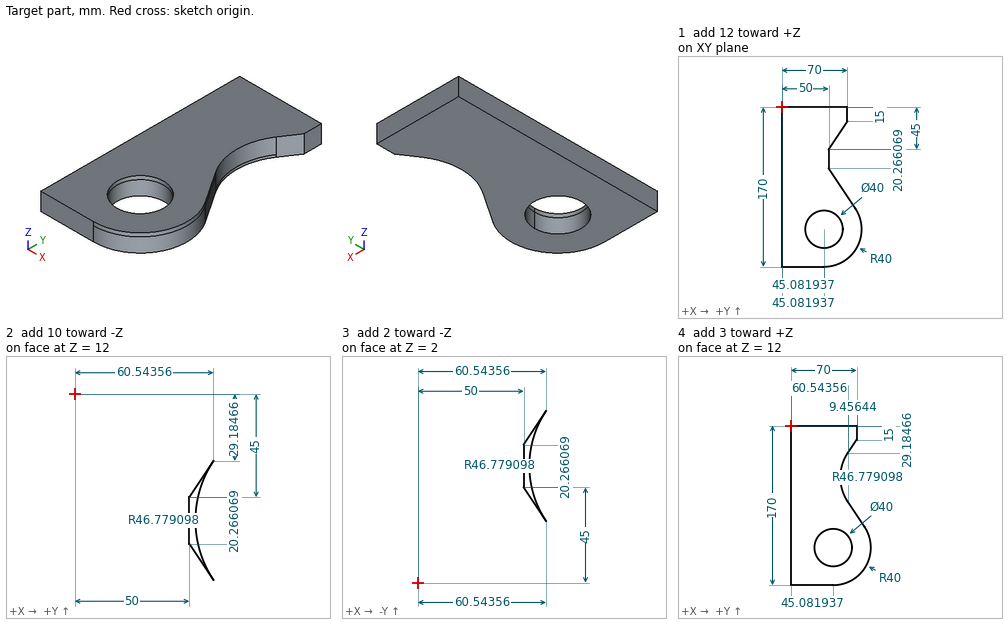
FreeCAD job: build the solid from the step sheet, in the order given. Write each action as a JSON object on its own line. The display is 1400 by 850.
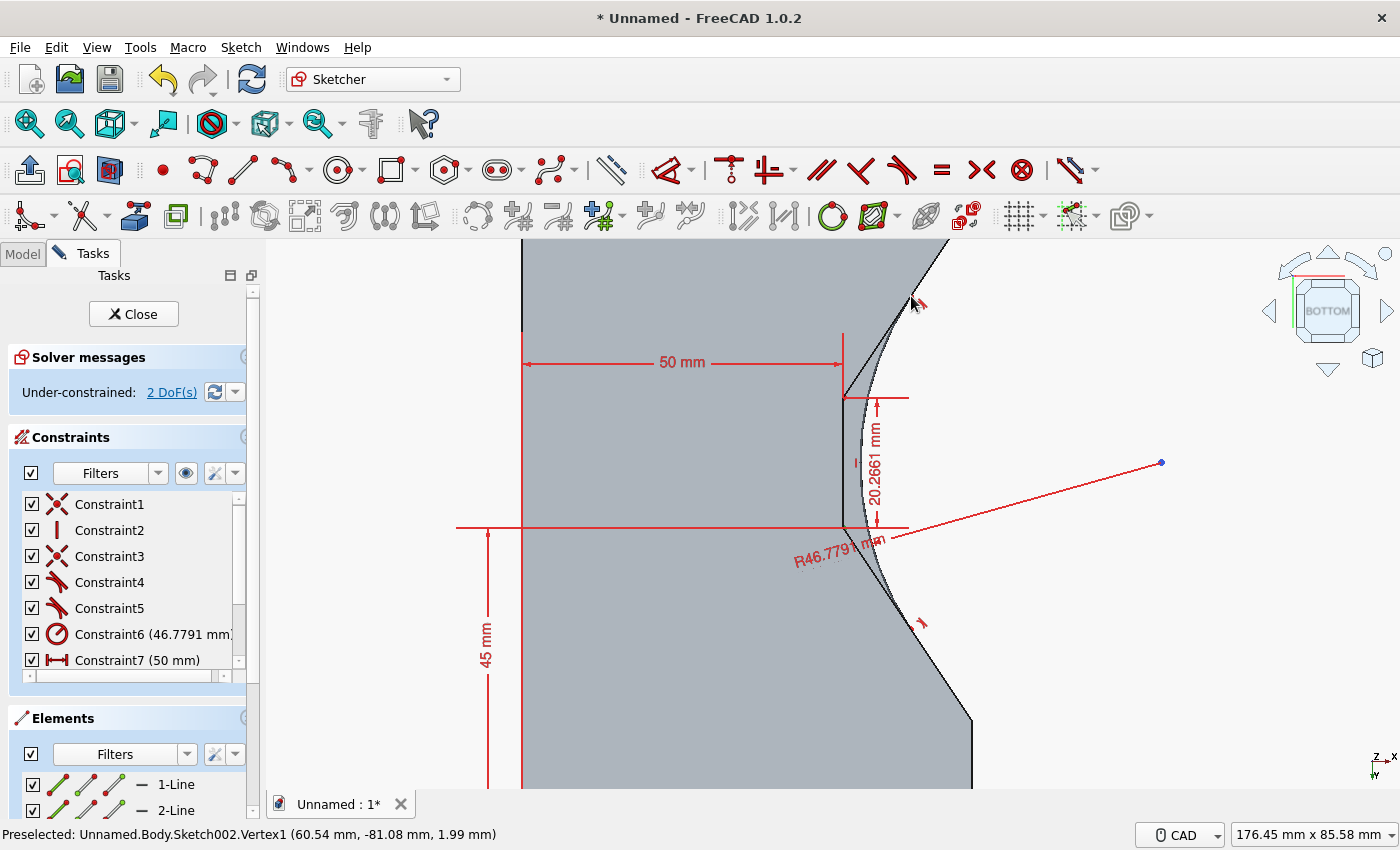
{"action": "left_click", "coordinate": [911, 296]}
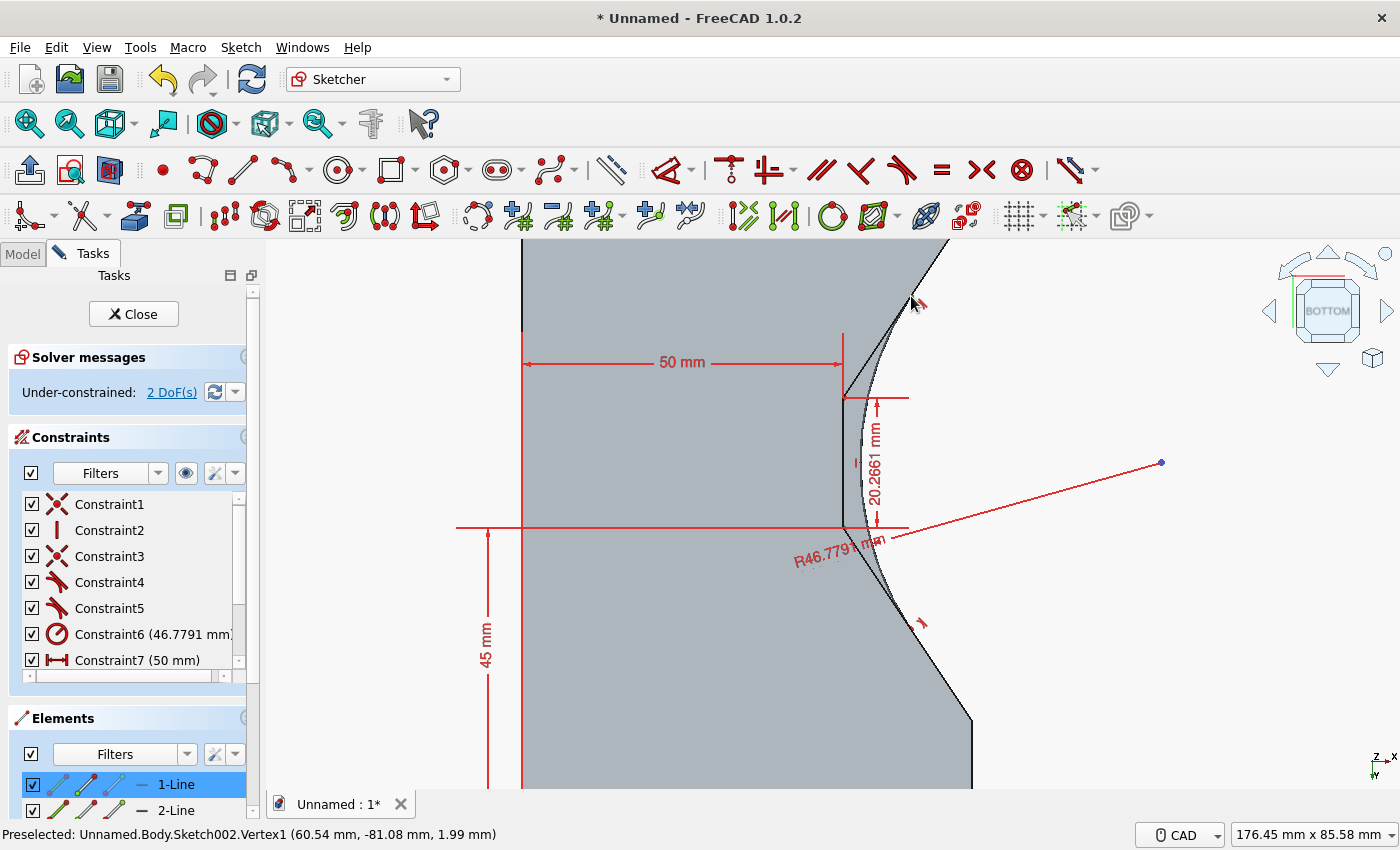
{"action": "key", "text": "l"}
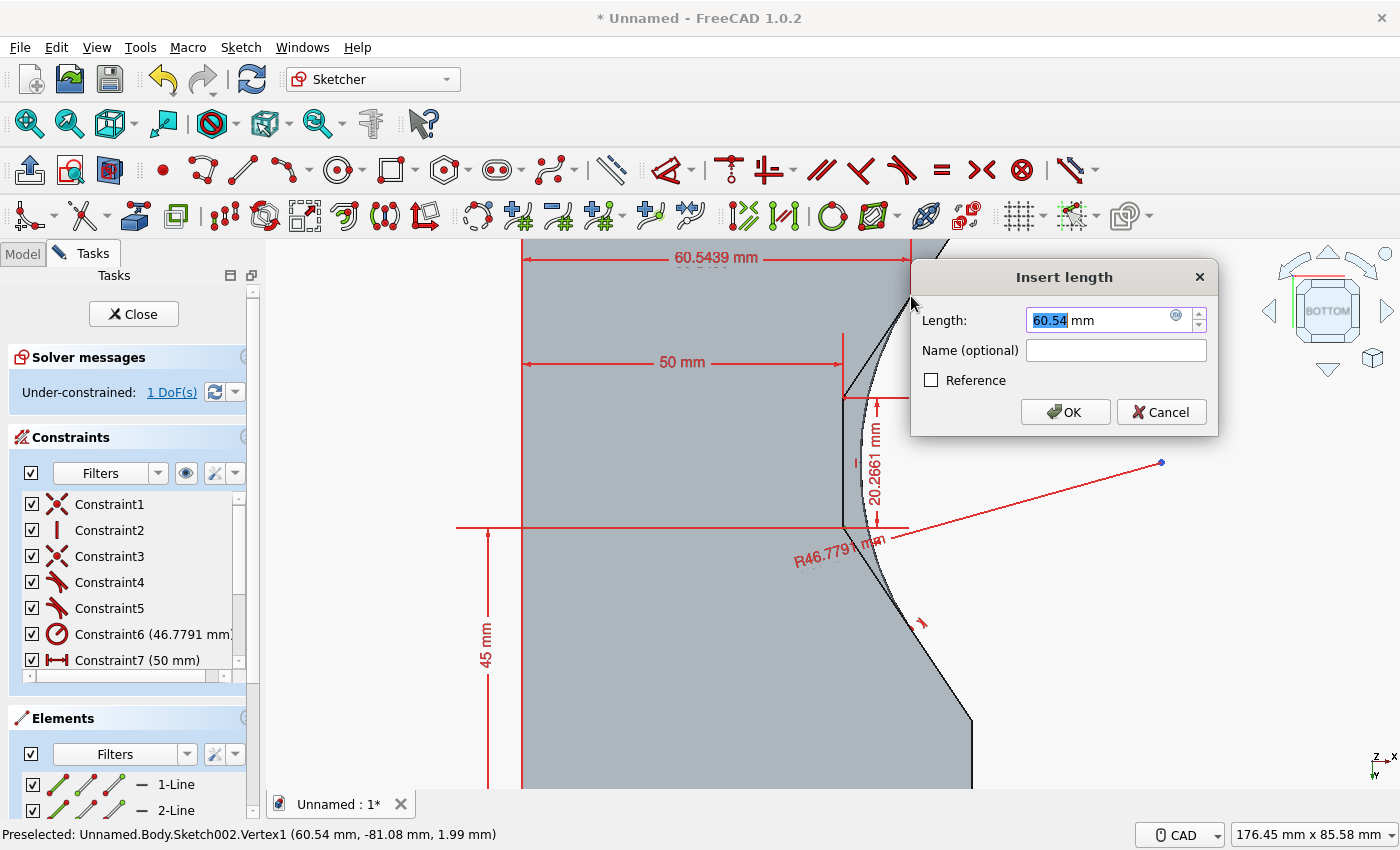
{"action": "type", "text": "60.54356"}
{"action": "key", "text": "Return"}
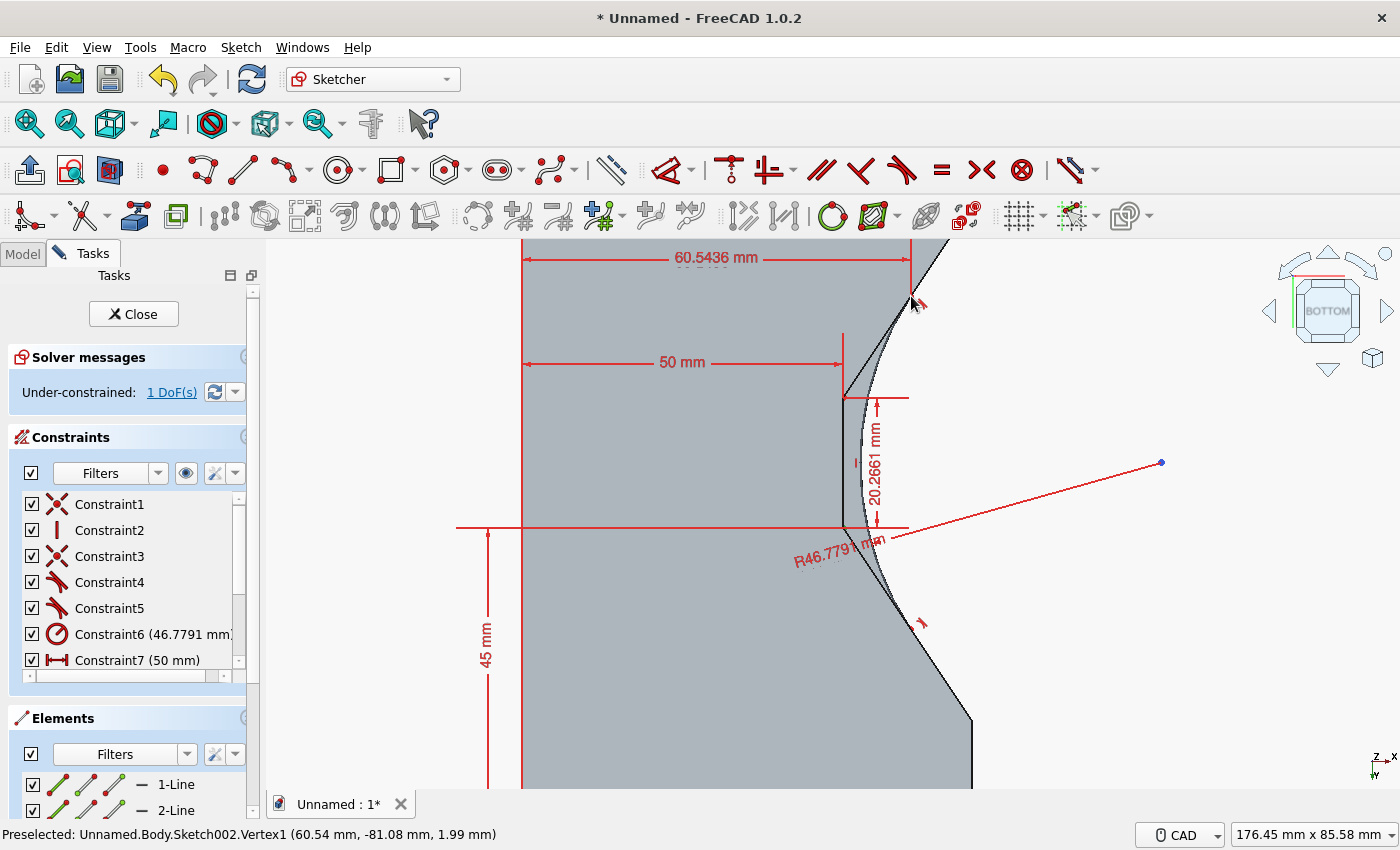
{"action": "left_click", "coordinate": [911, 630]}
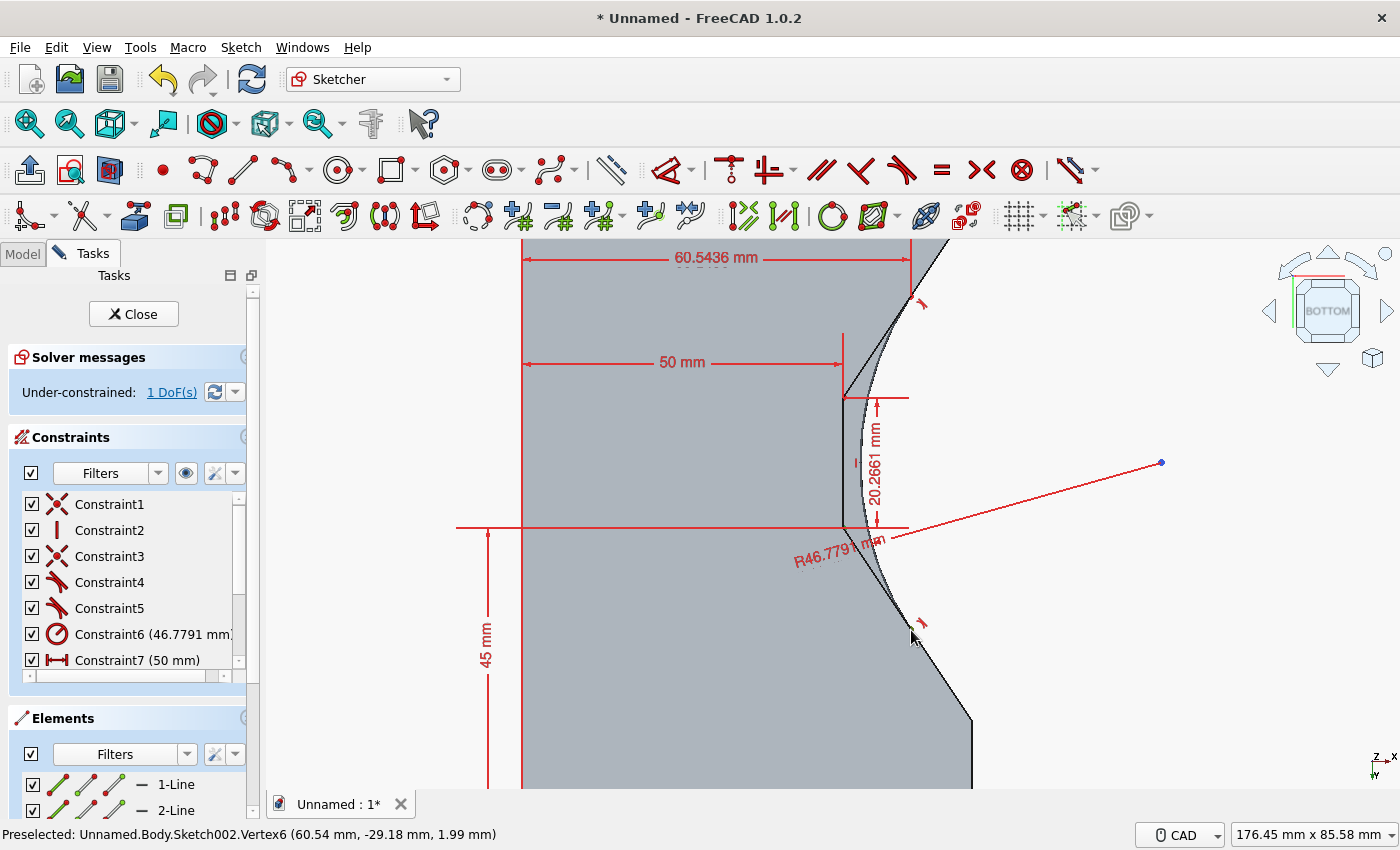
{"action": "key", "text": "l"}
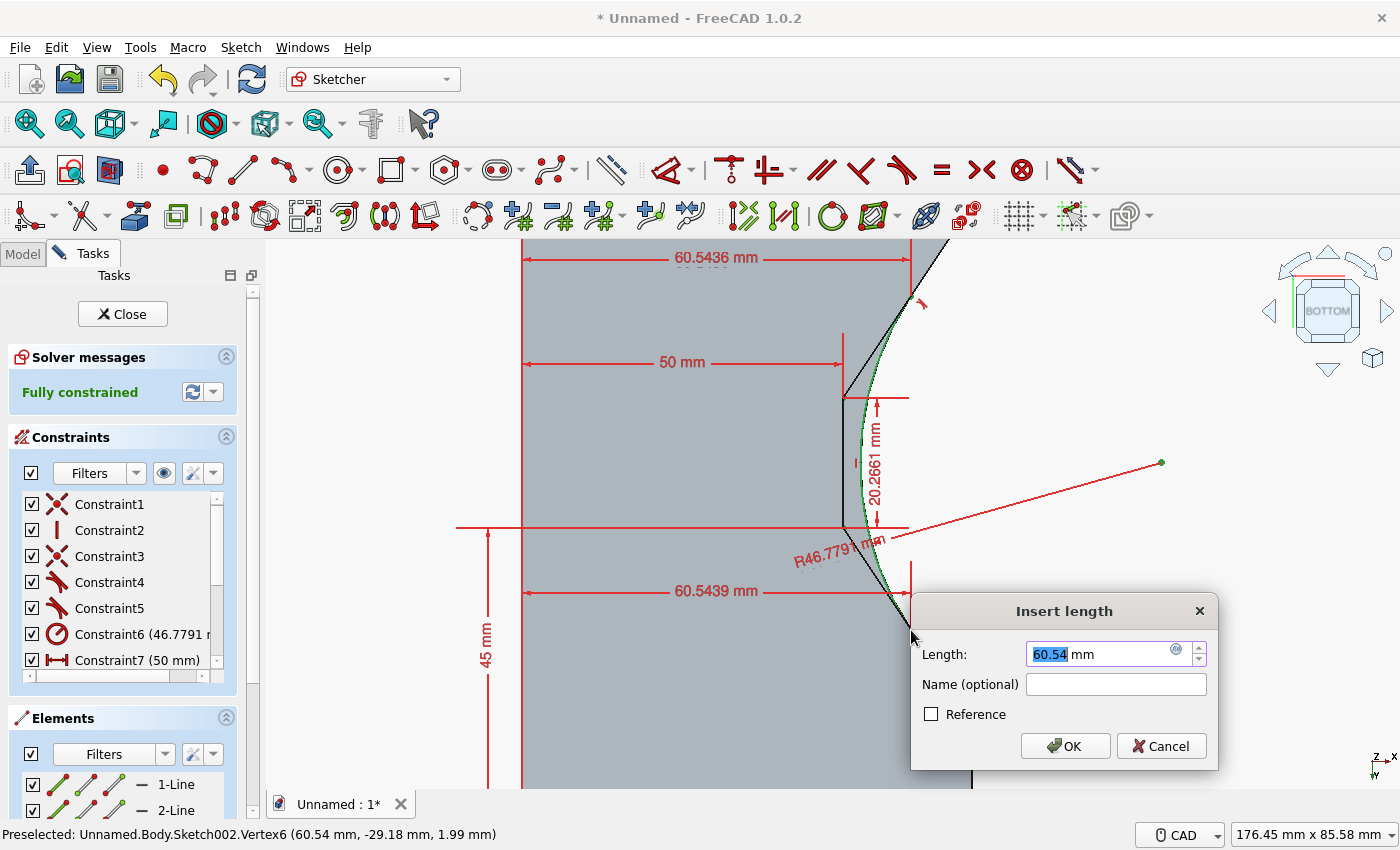
{"action": "type", "text": "60.54356"}
{"action": "key", "text": "Return"}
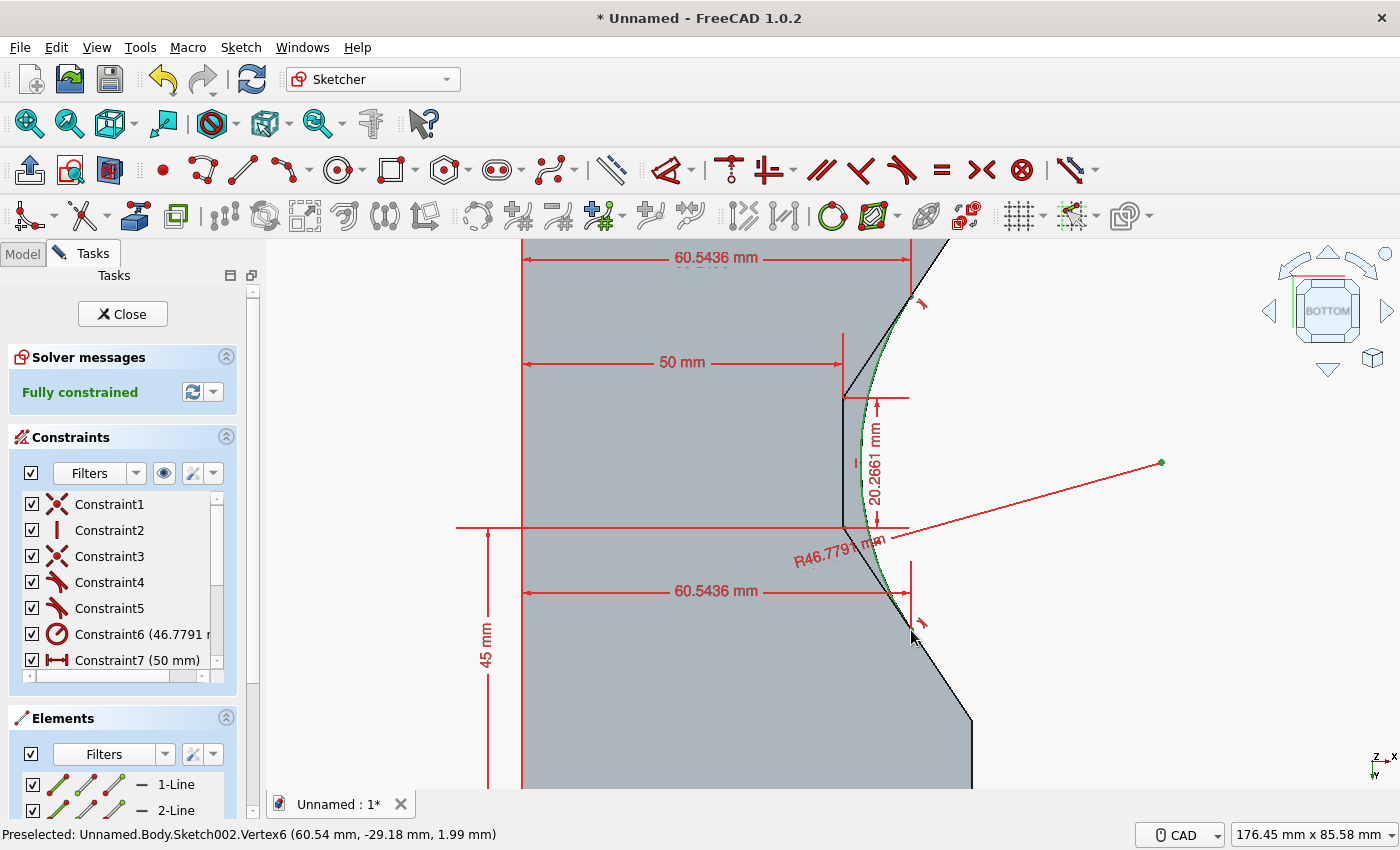
{"action": "left_click", "coordinate": [123, 314]}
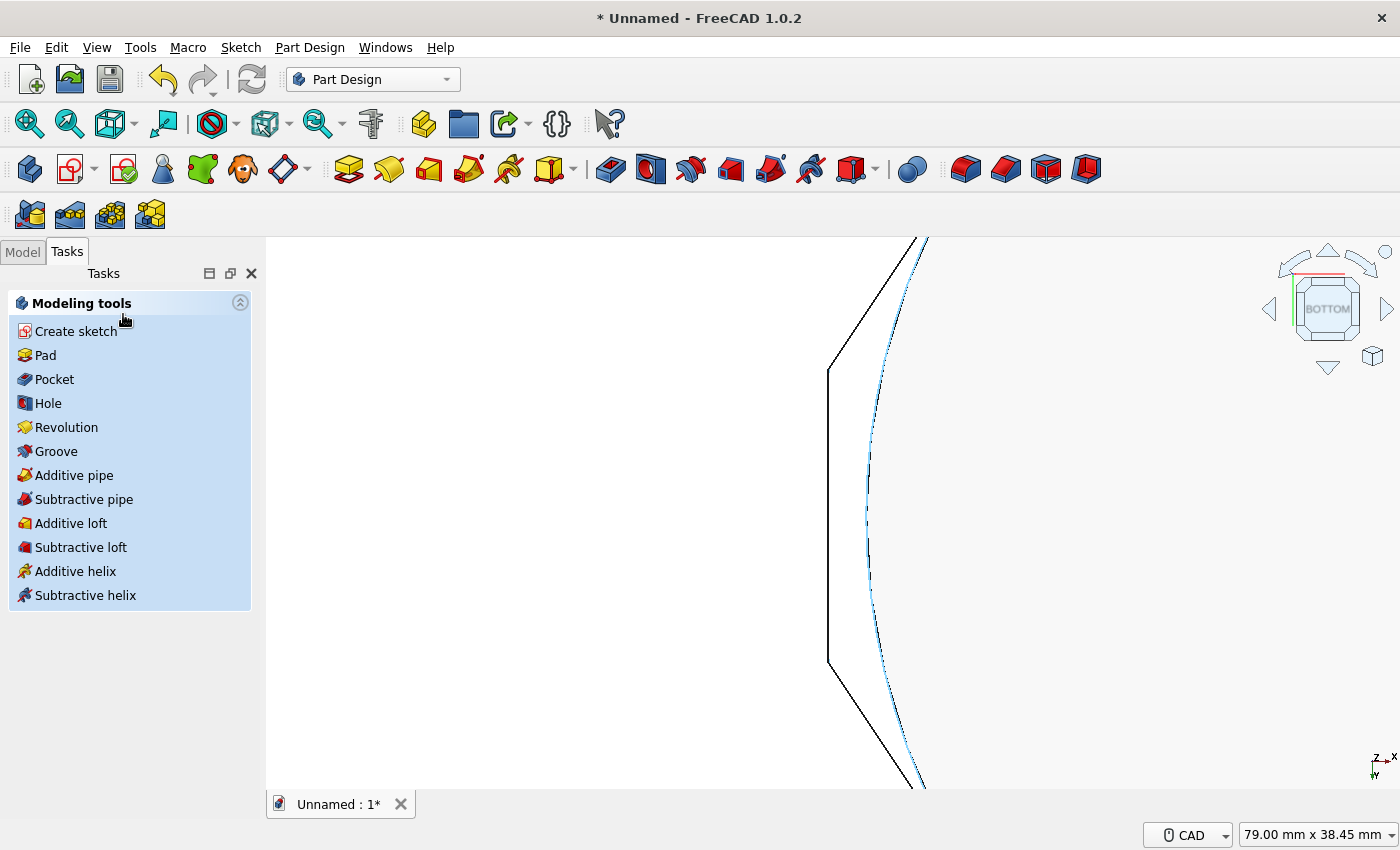
{"action": "left_click", "coordinate": [350, 170]}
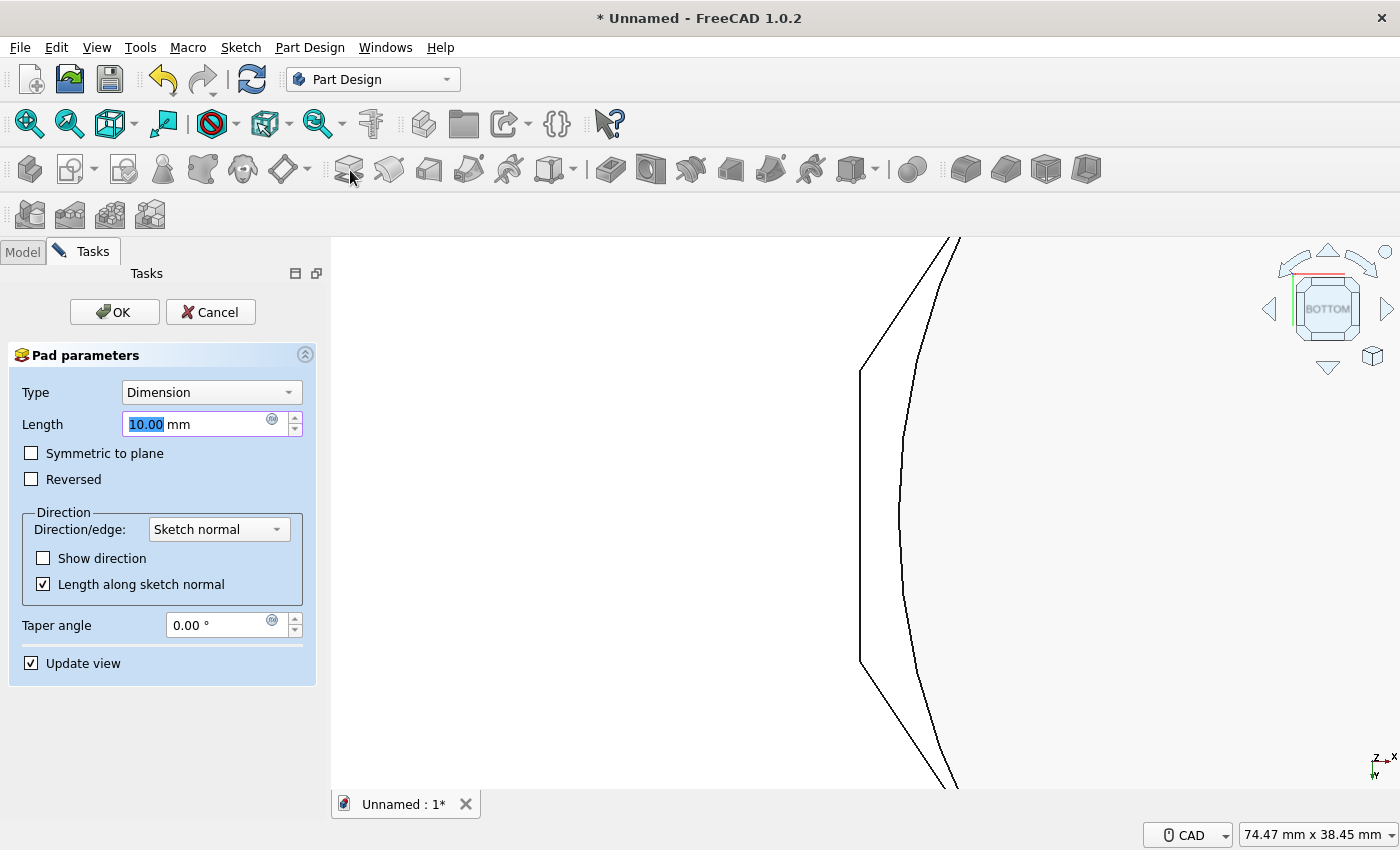
{"action": "type", "text": "2"}
{"action": "key", "text": "Tab"}